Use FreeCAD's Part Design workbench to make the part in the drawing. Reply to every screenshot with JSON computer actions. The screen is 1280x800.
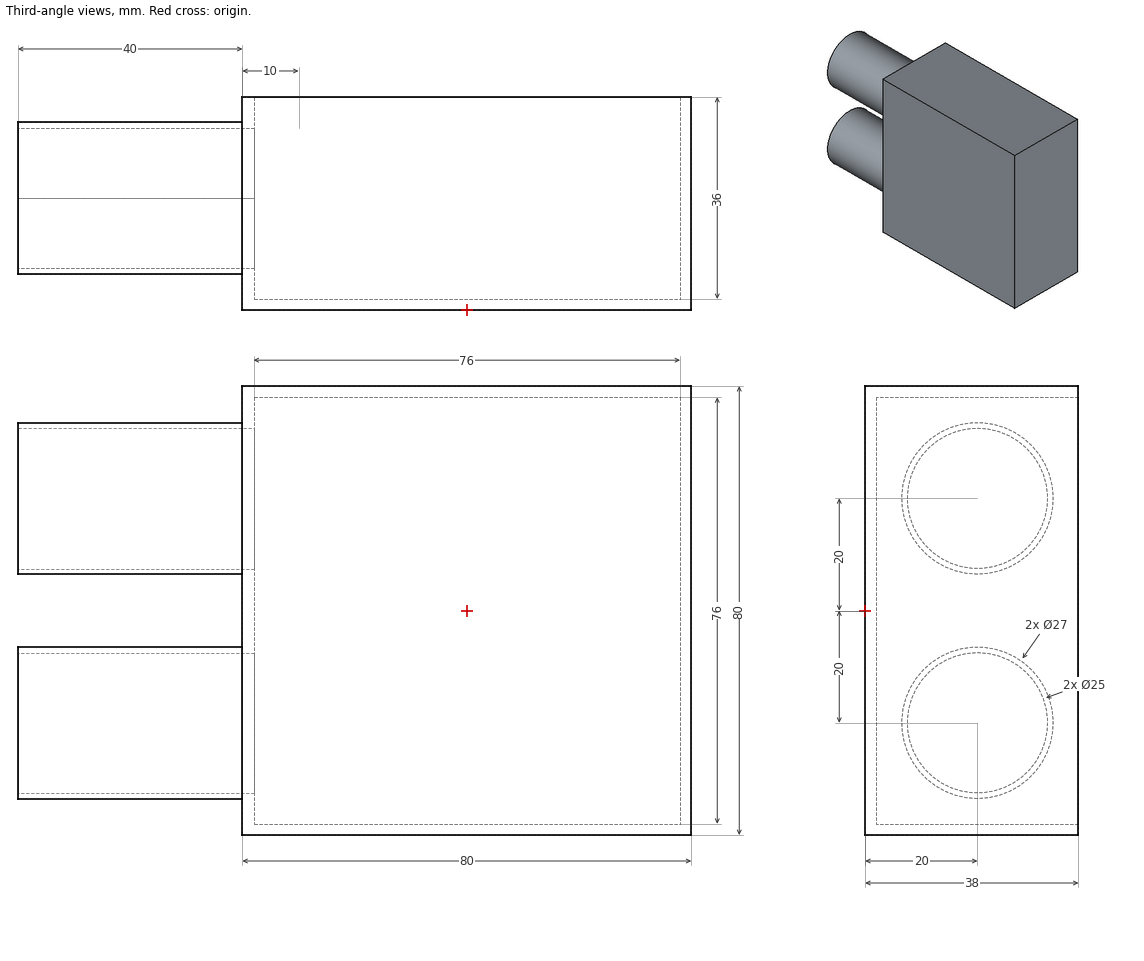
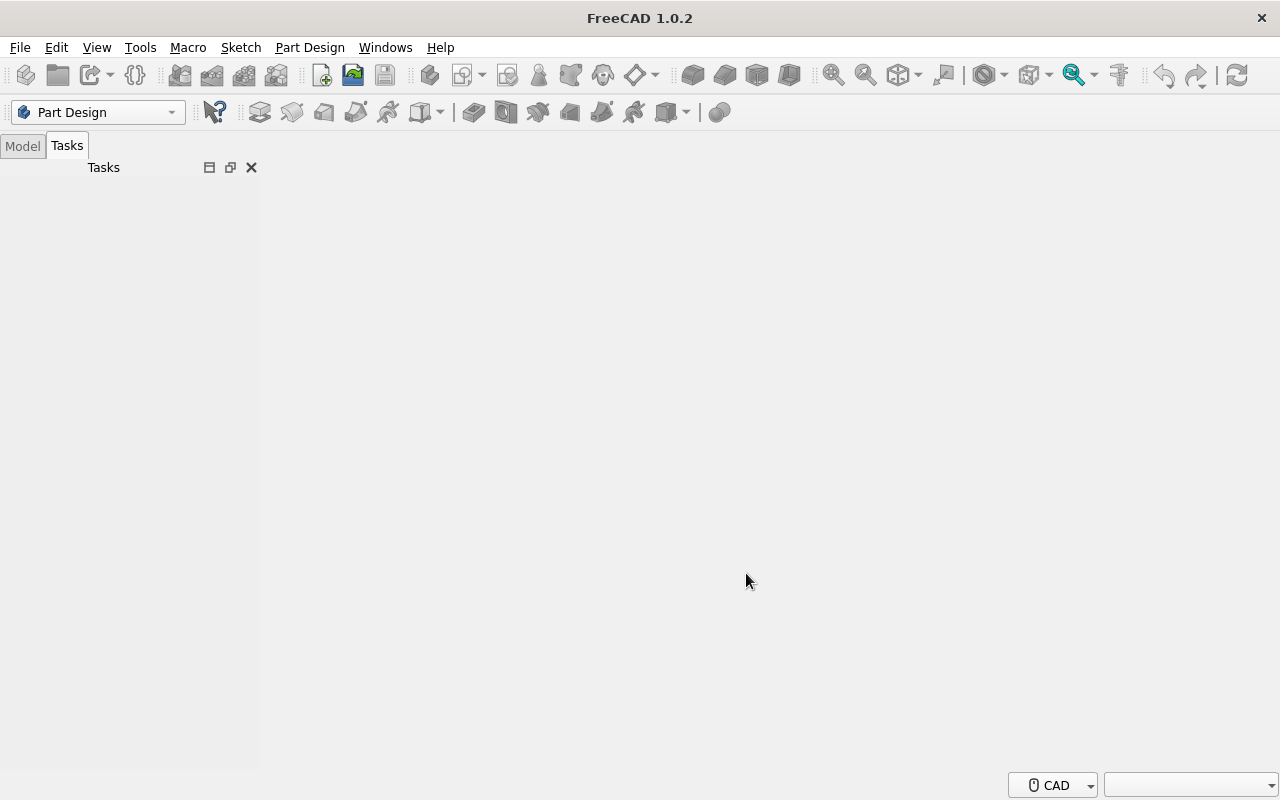
{"action": "left_click", "coordinate": [322, 76]}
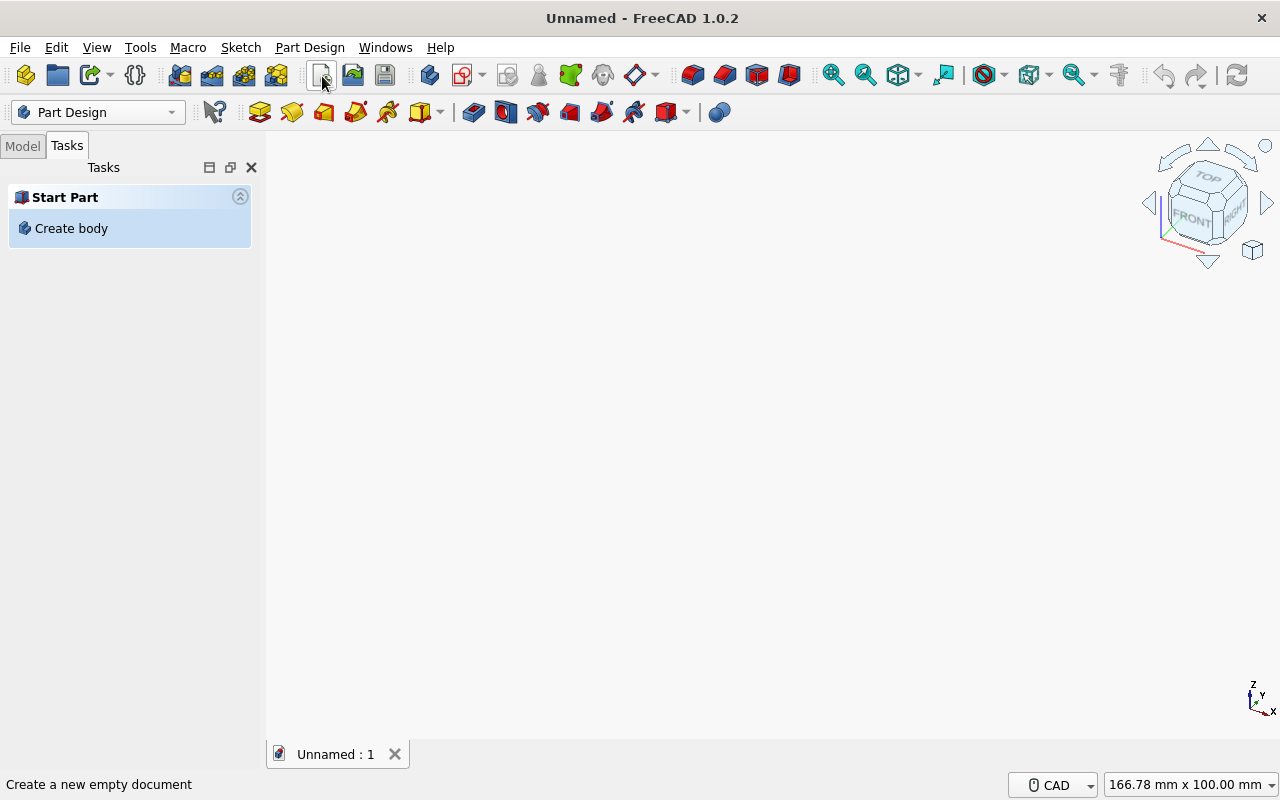
{"action": "left_click", "coordinate": [462, 76]}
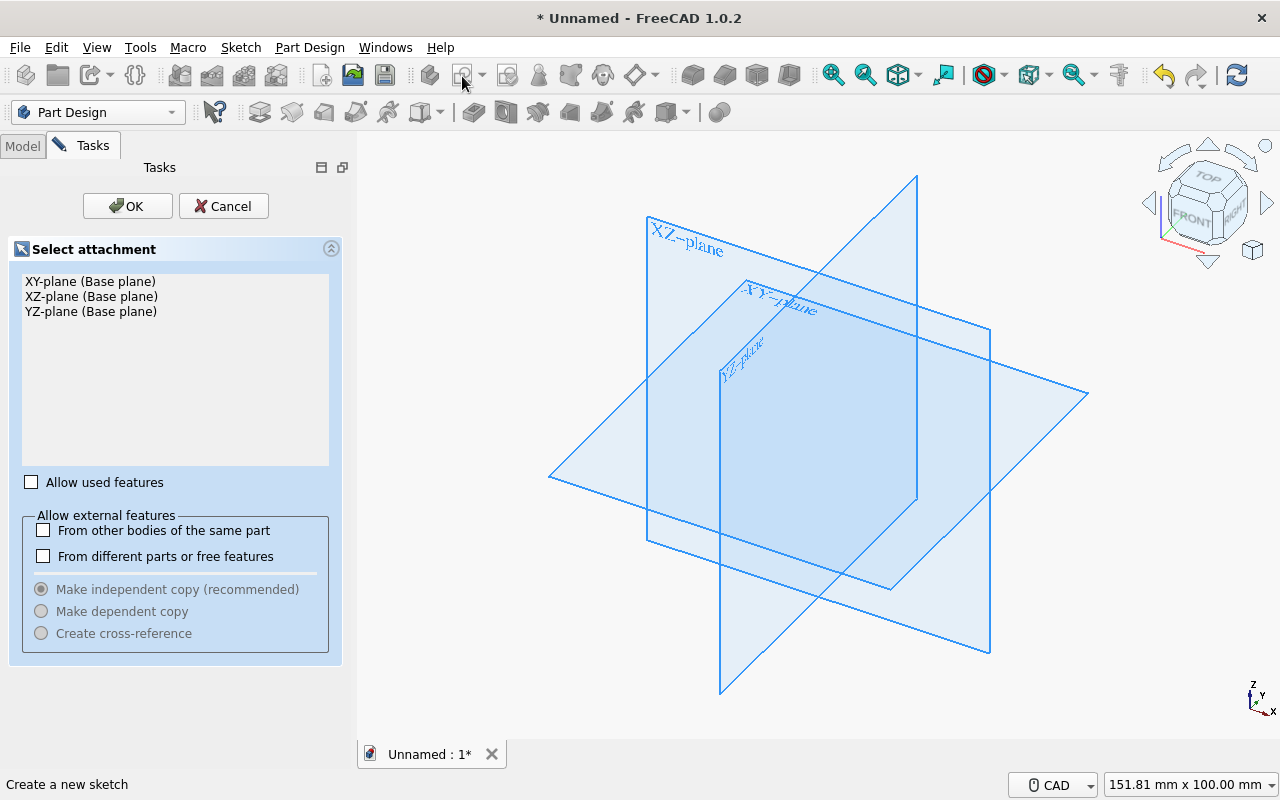
{"action": "left_click", "coordinate": [82, 296]}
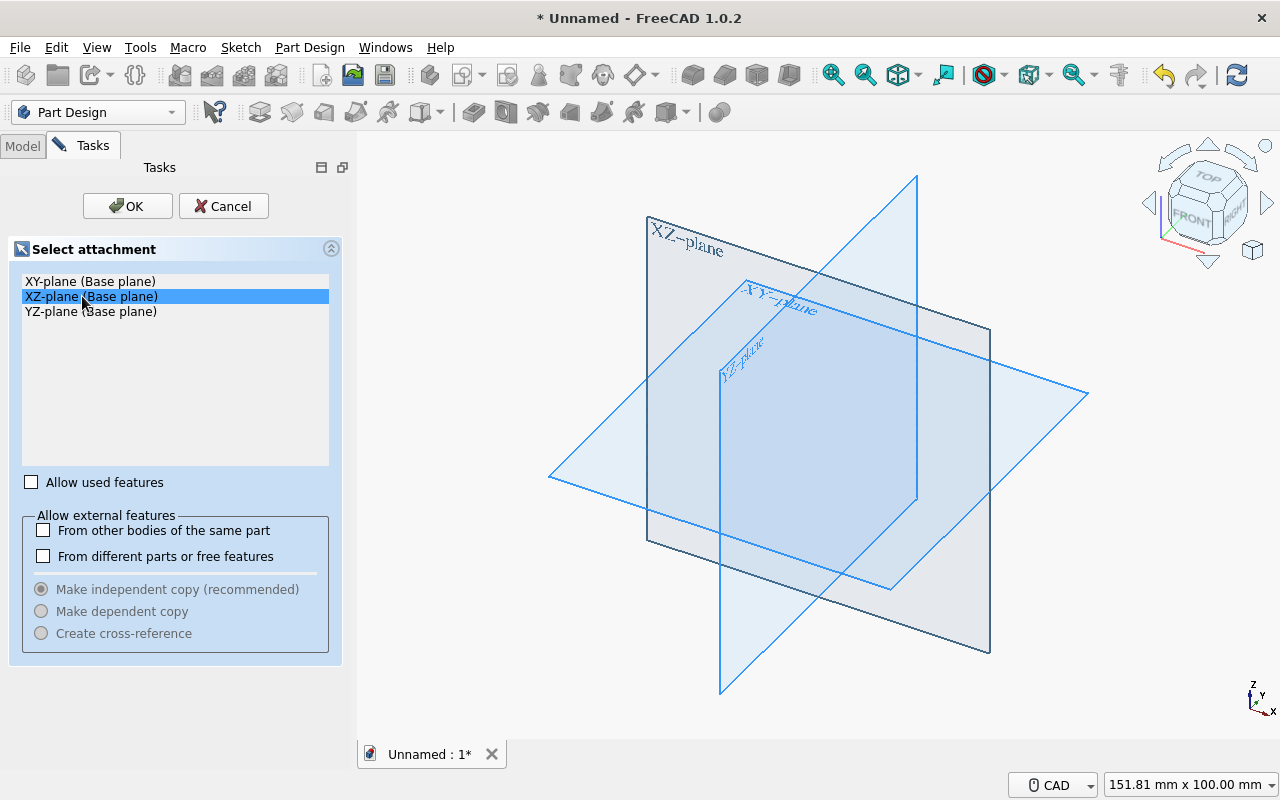
{"action": "left_click", "coordinate": [128, 206]}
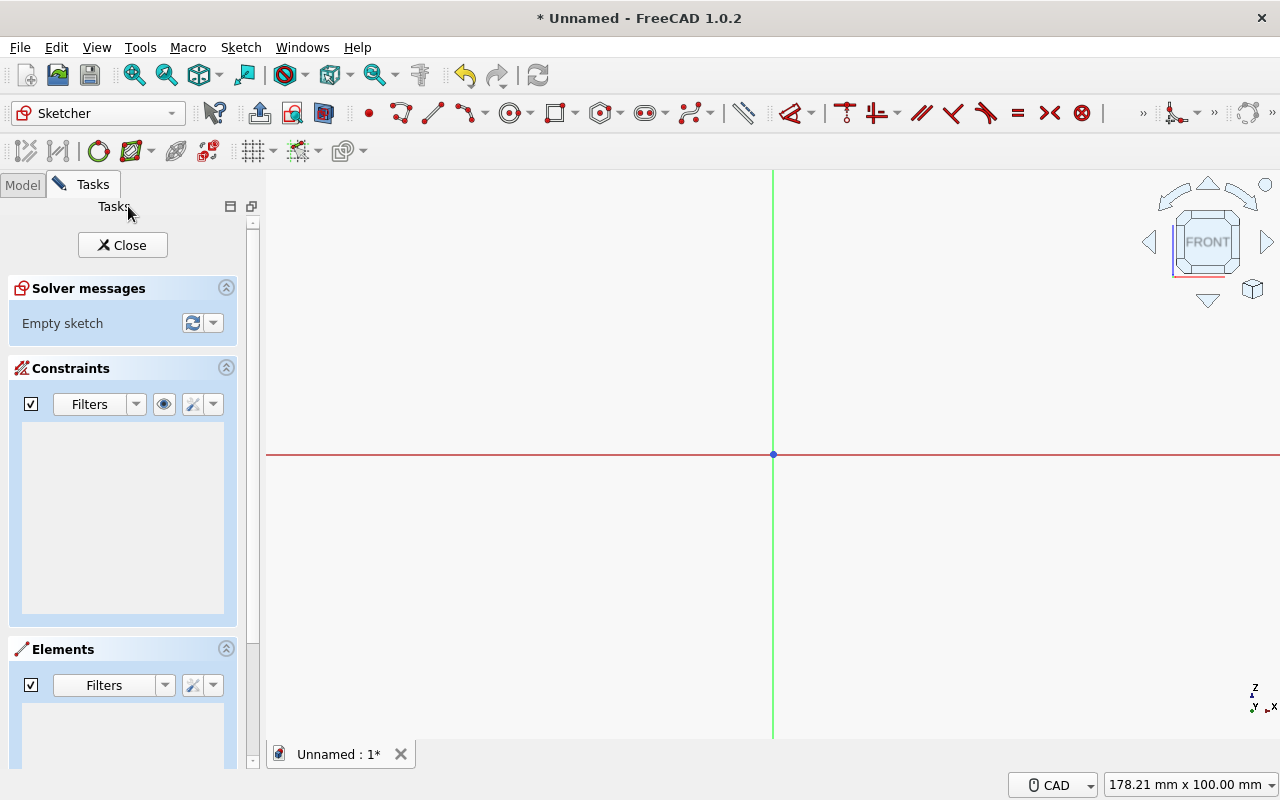
{"action": "key", "text": "g v"}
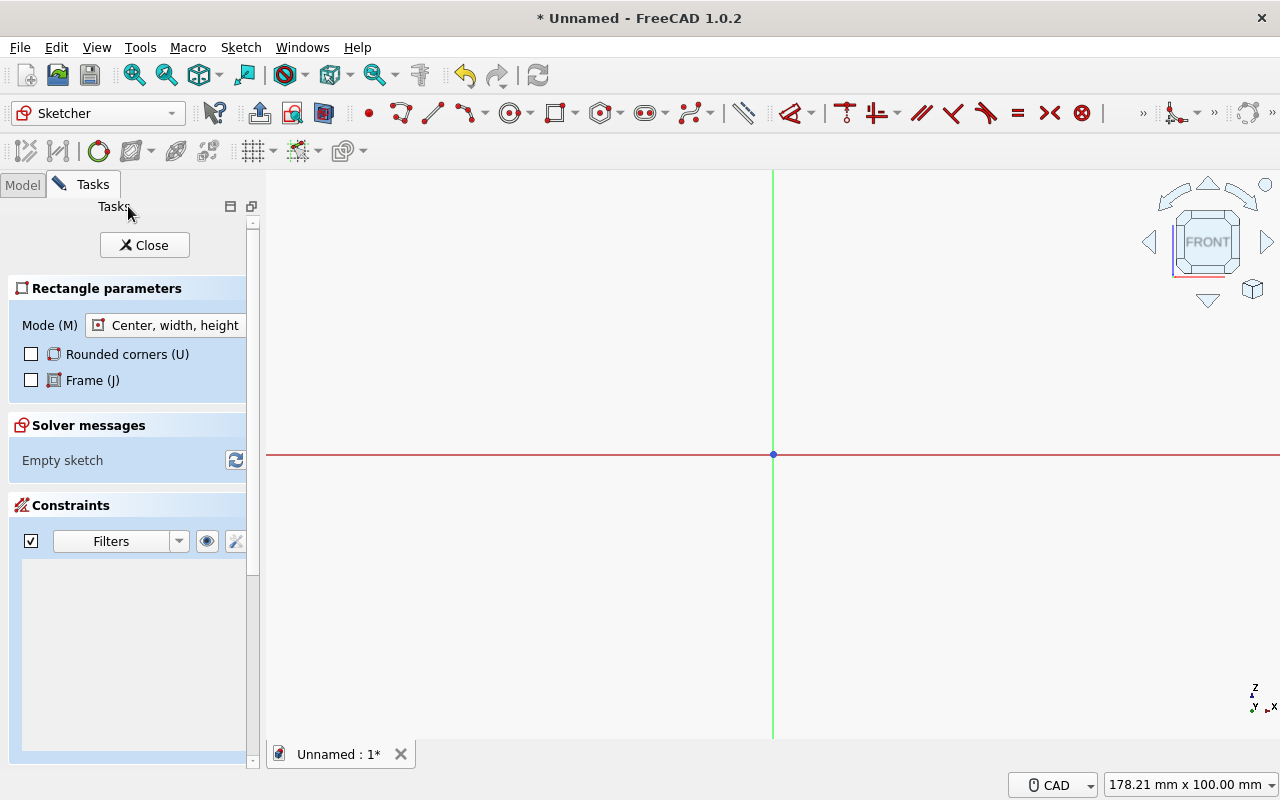
{"action": "left_click", "coordinate": [773, 454]}
{"action": "mouse_move", "coordinate": [1001, 227]}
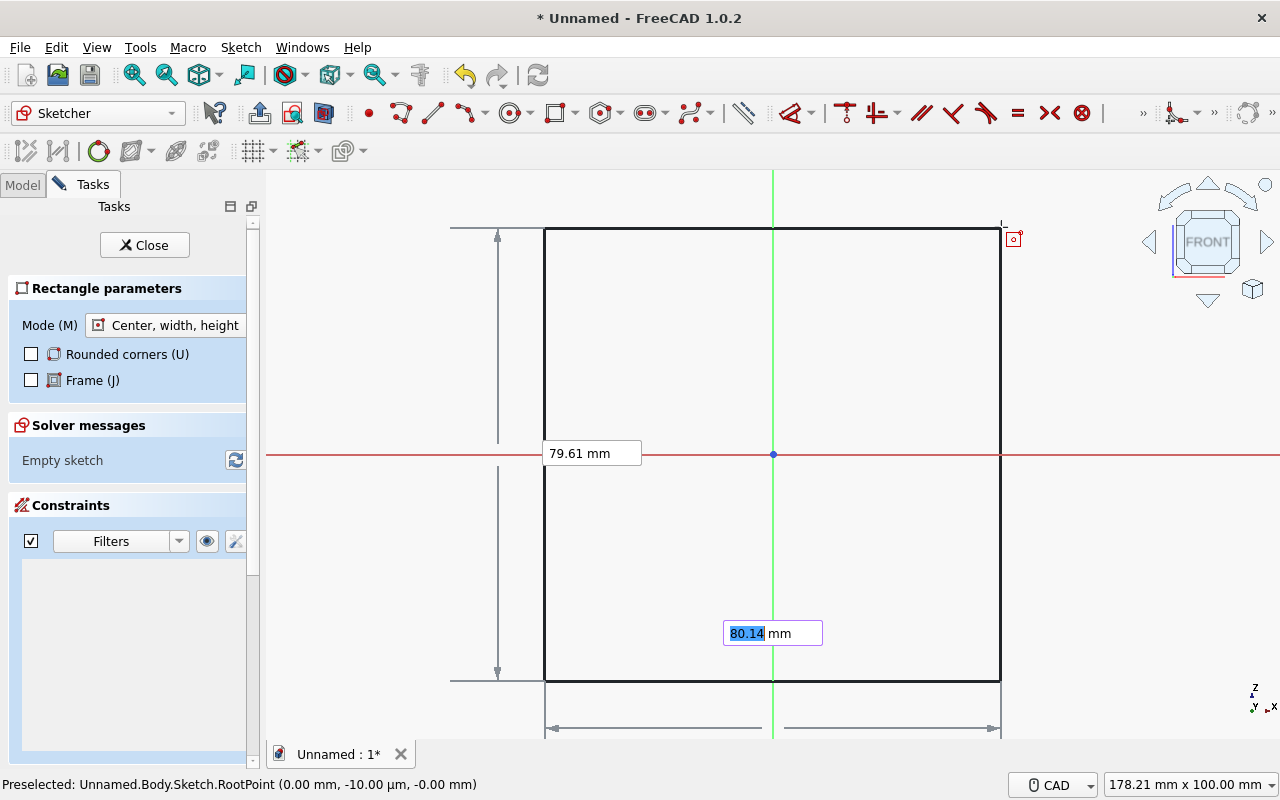
{"action": "type", "text": "80"}
{"action": "key", "text": "Tab"}
{"action": "type", "text": "80"}
{"action": "key", "text": "Return"}
{"action": "key", "text": "Escape"}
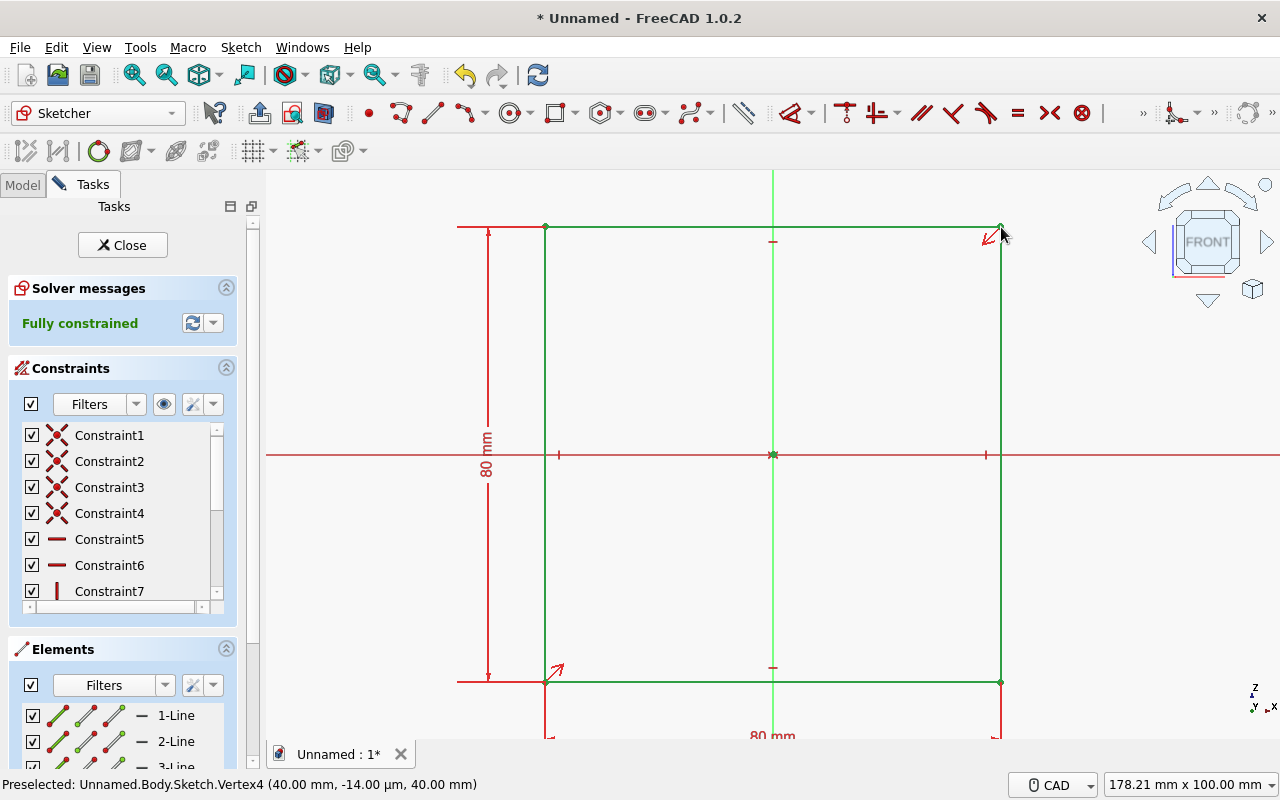
{"action": "left_click", "coordinate": [123, 245]}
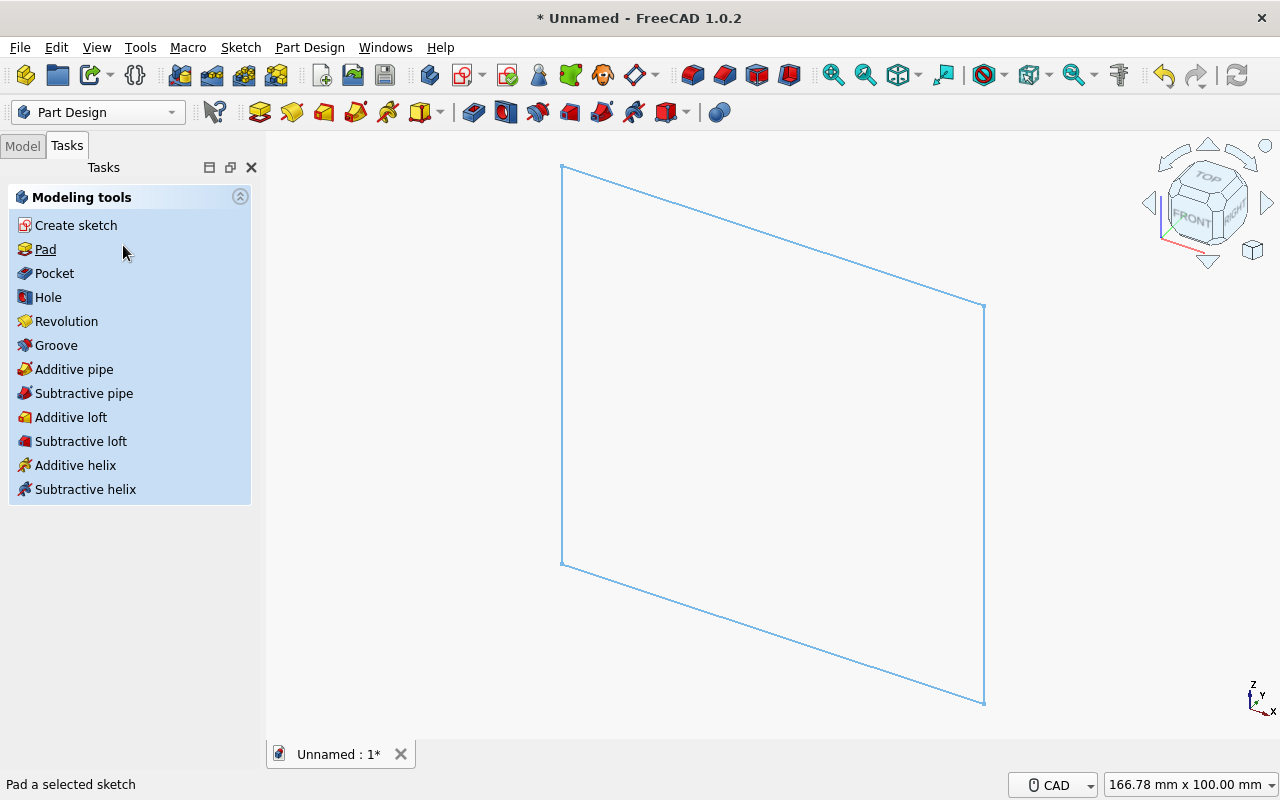
{"action": "left_click", "coordinate": [260, 112]}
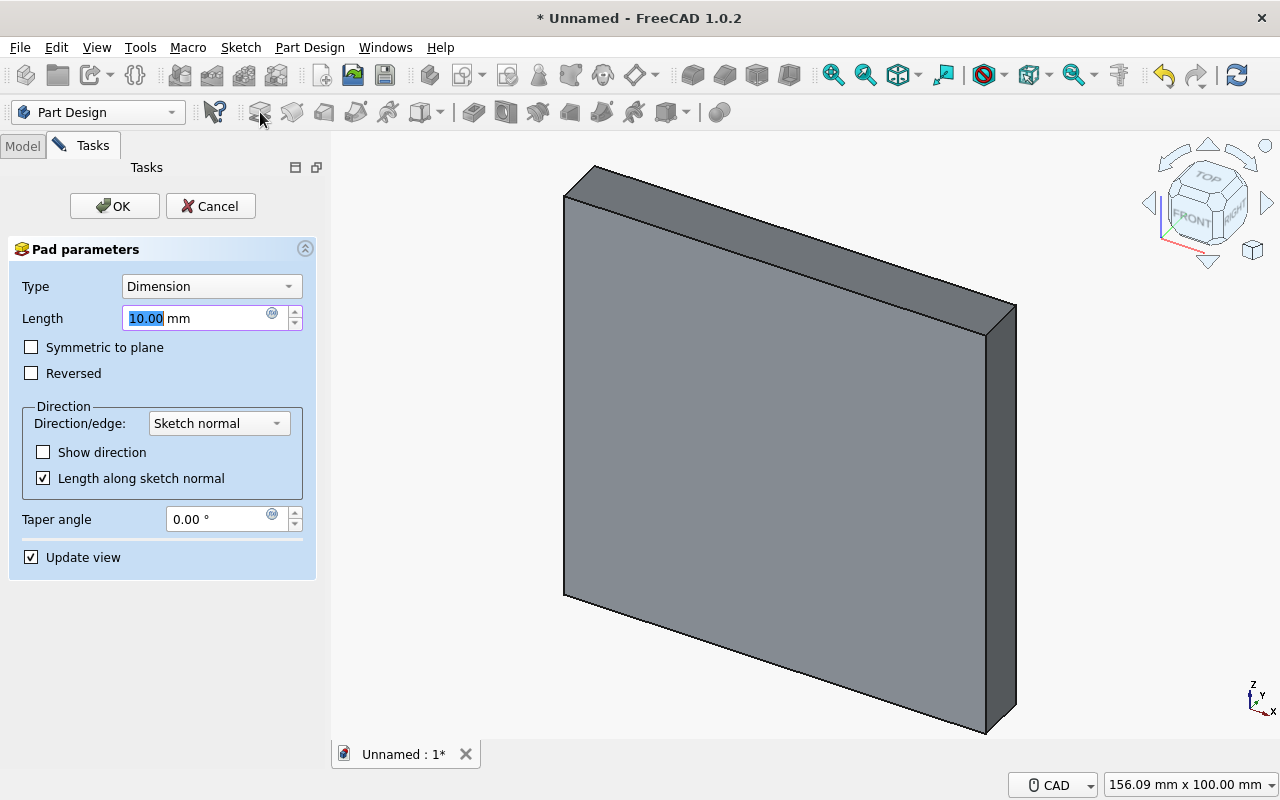
{"action": "type", "text": "38"}
{"action": "key", "text": "Tab"}